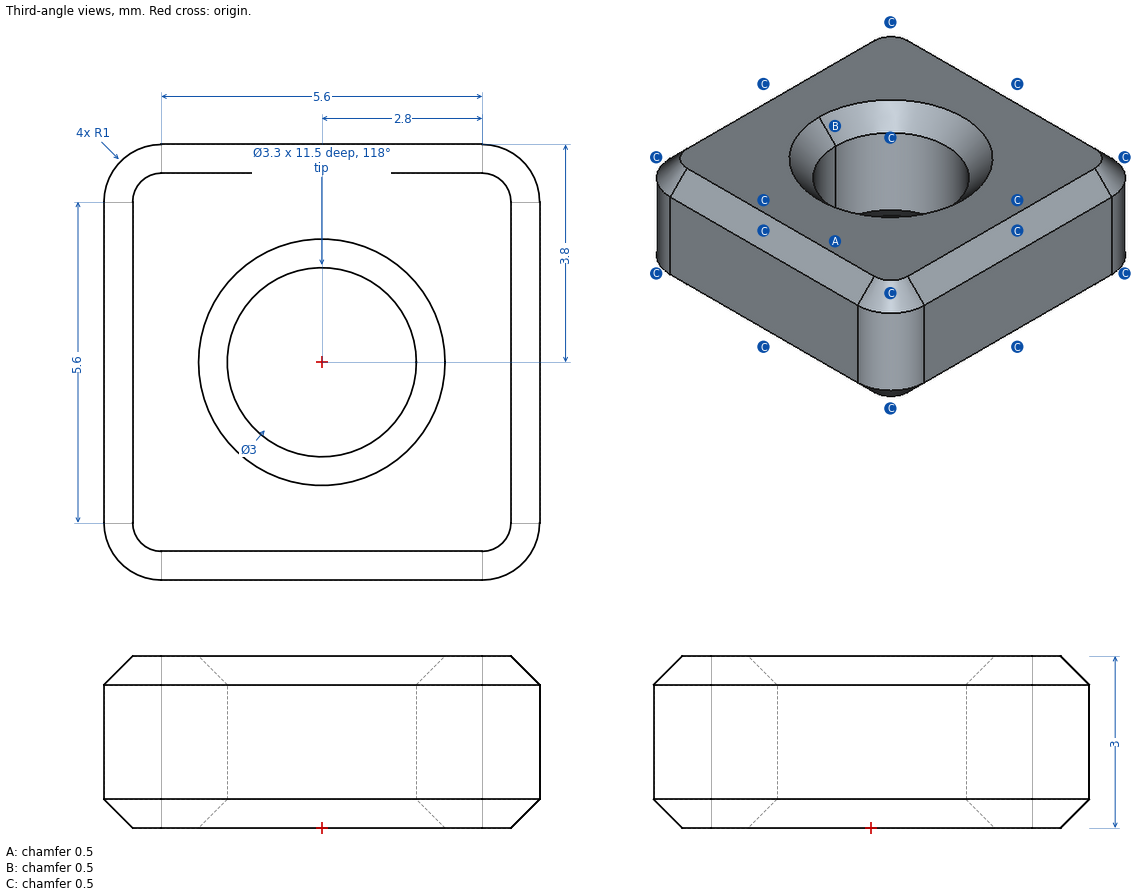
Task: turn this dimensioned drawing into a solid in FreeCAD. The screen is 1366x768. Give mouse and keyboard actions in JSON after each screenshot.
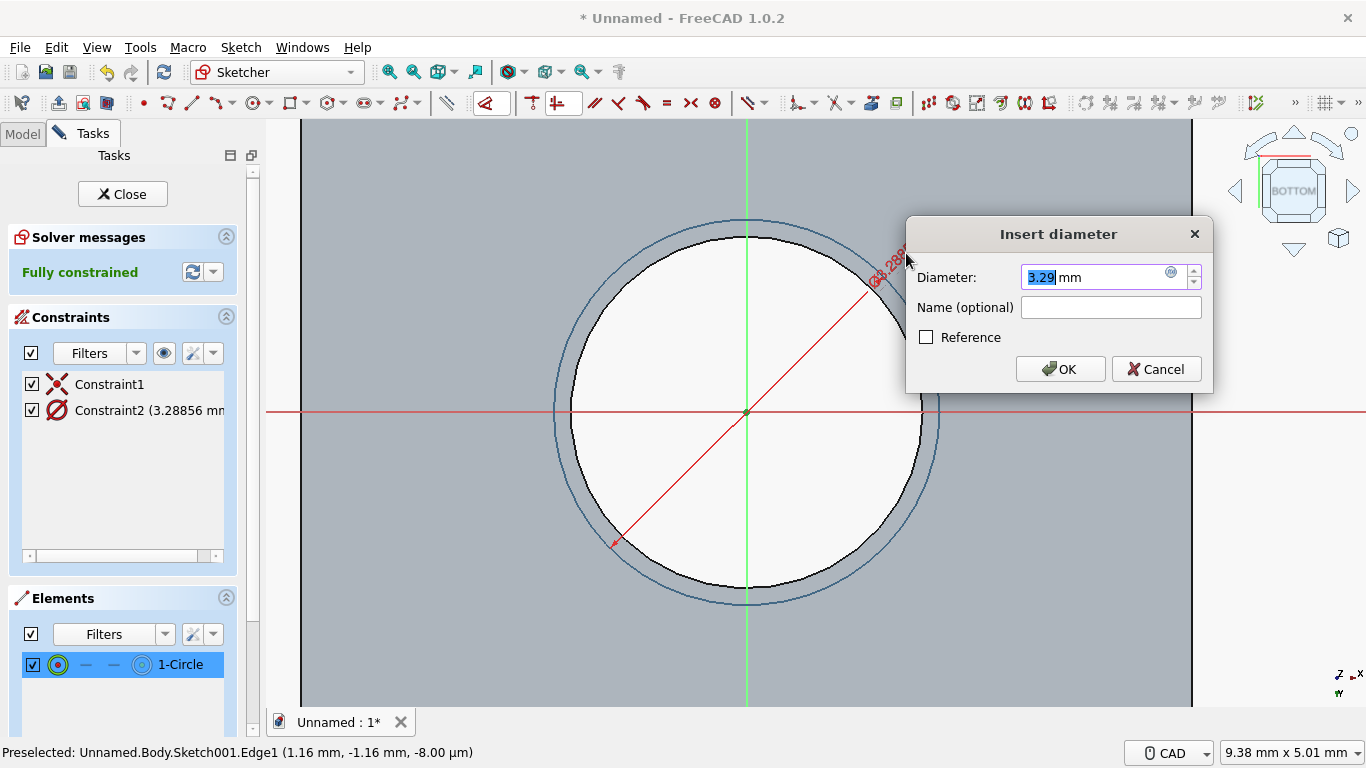
{"action": "type", "text": "3.3"}
{"action": "key", "text": "Return"}
{"action": "key", "text": "Escape"}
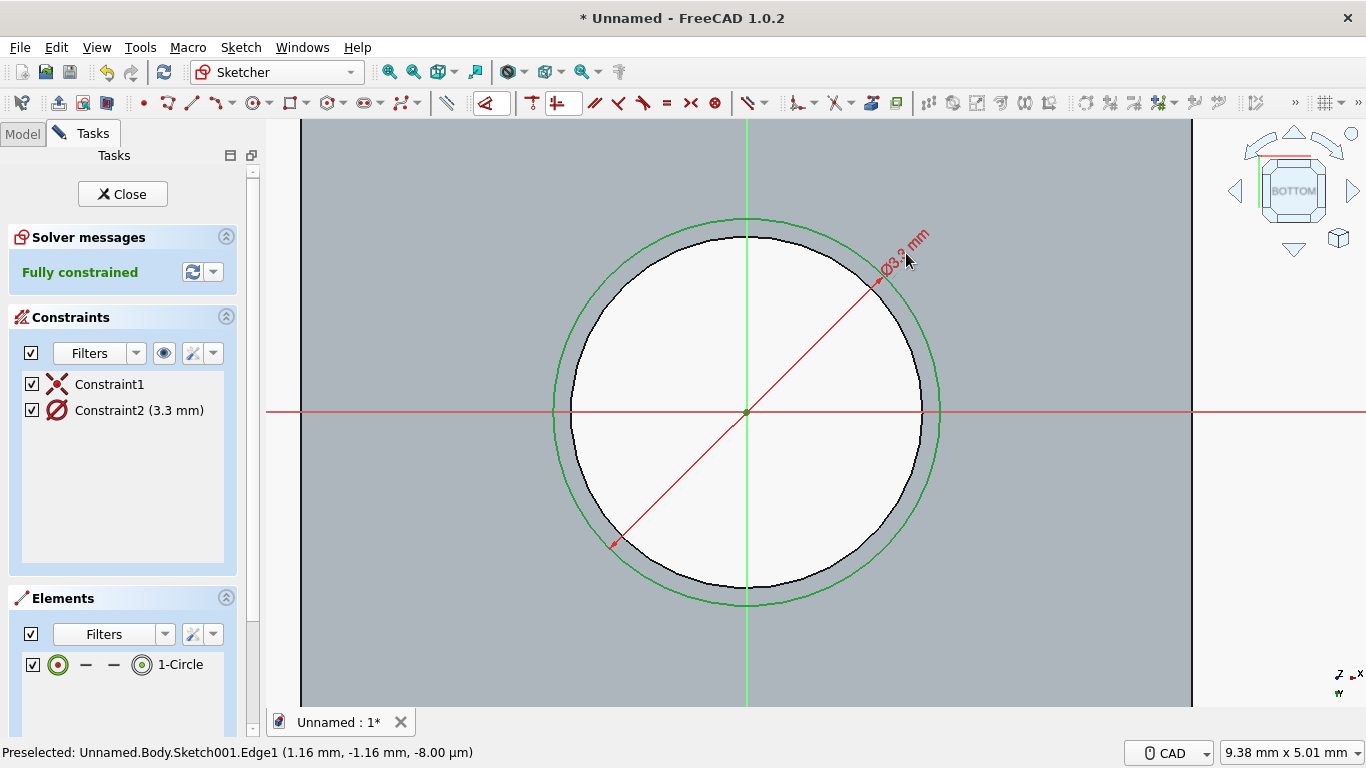
{"action": "left_click", "coordinate": [123, 194]}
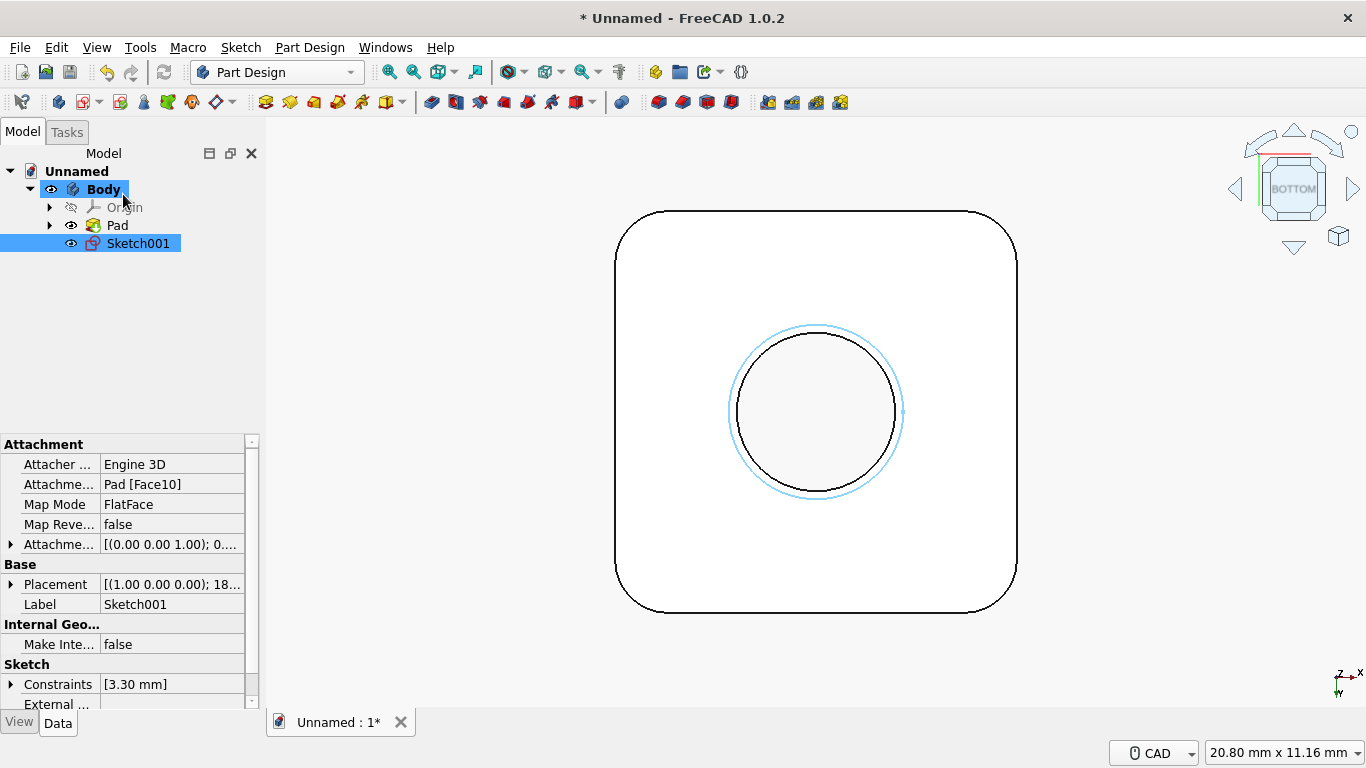
{"action": "left_click", "coordinate": [456, 102]}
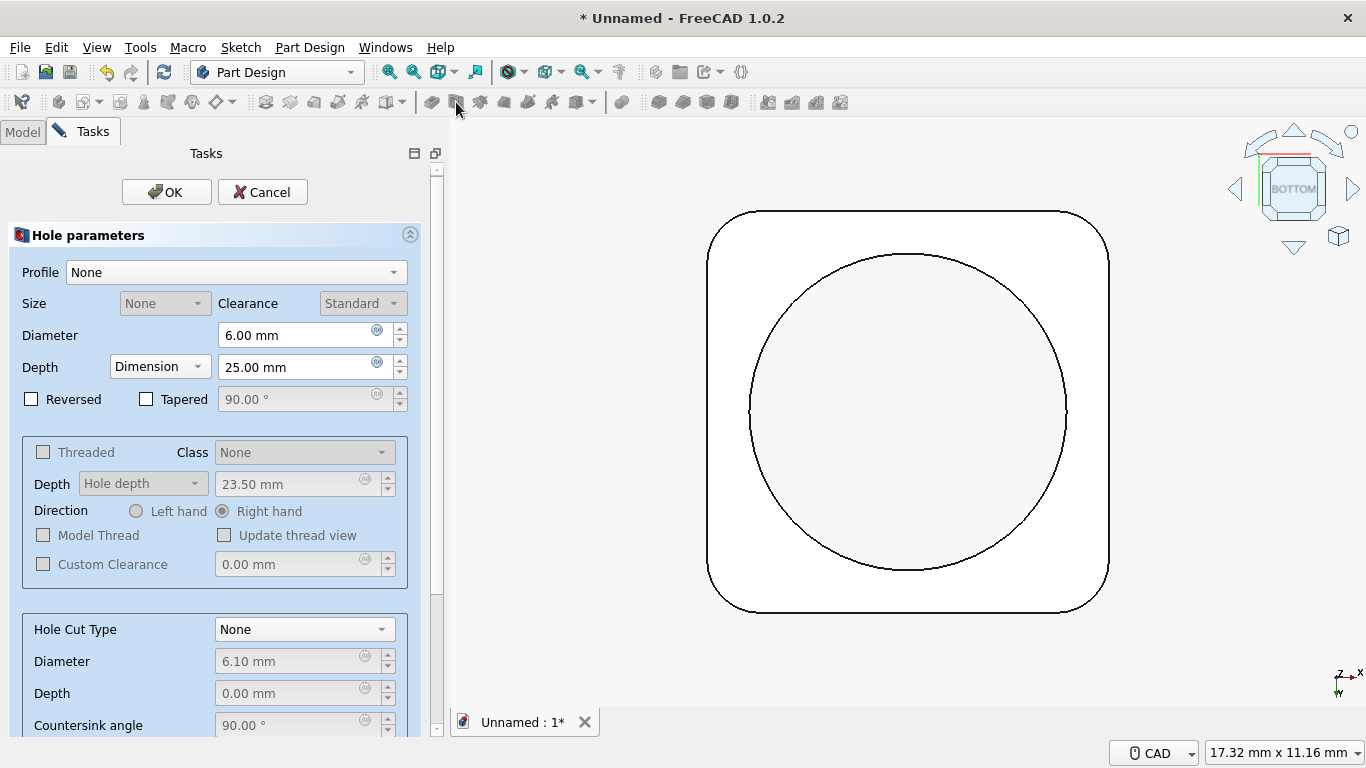
{"action": "triple_click", "coordinate": [305, 335]}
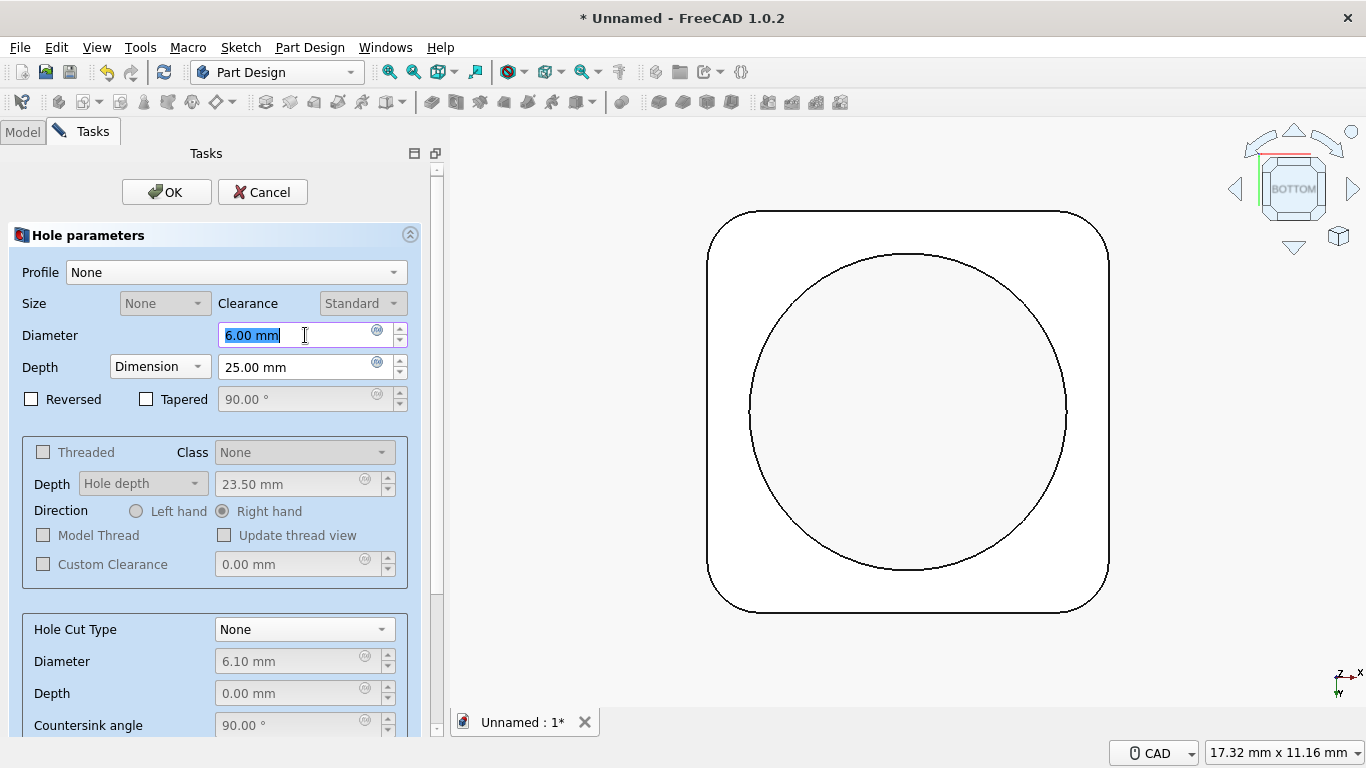
{"action": "type", "text": "3.3"}
{"action": "key", "text": "Tab"}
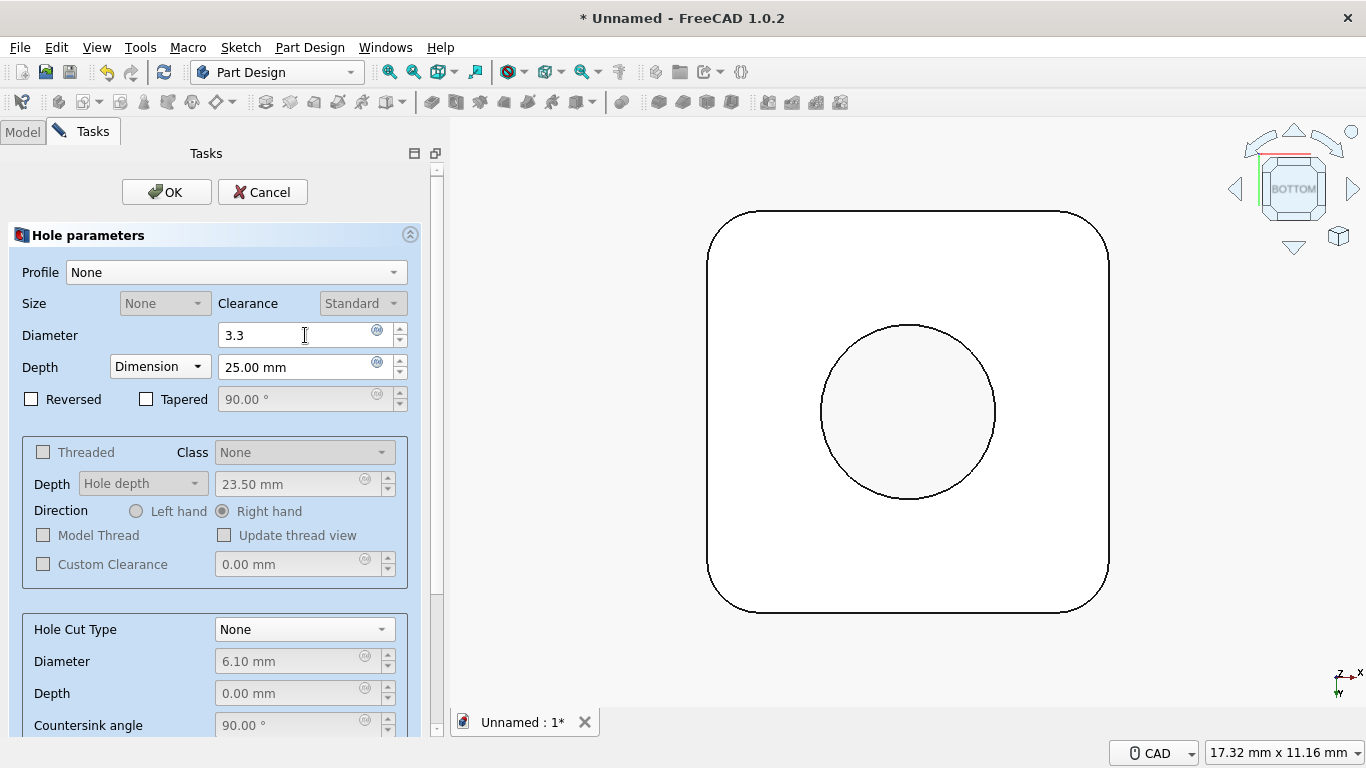
{"action": "triple_click", "coordinate": [305, 367]}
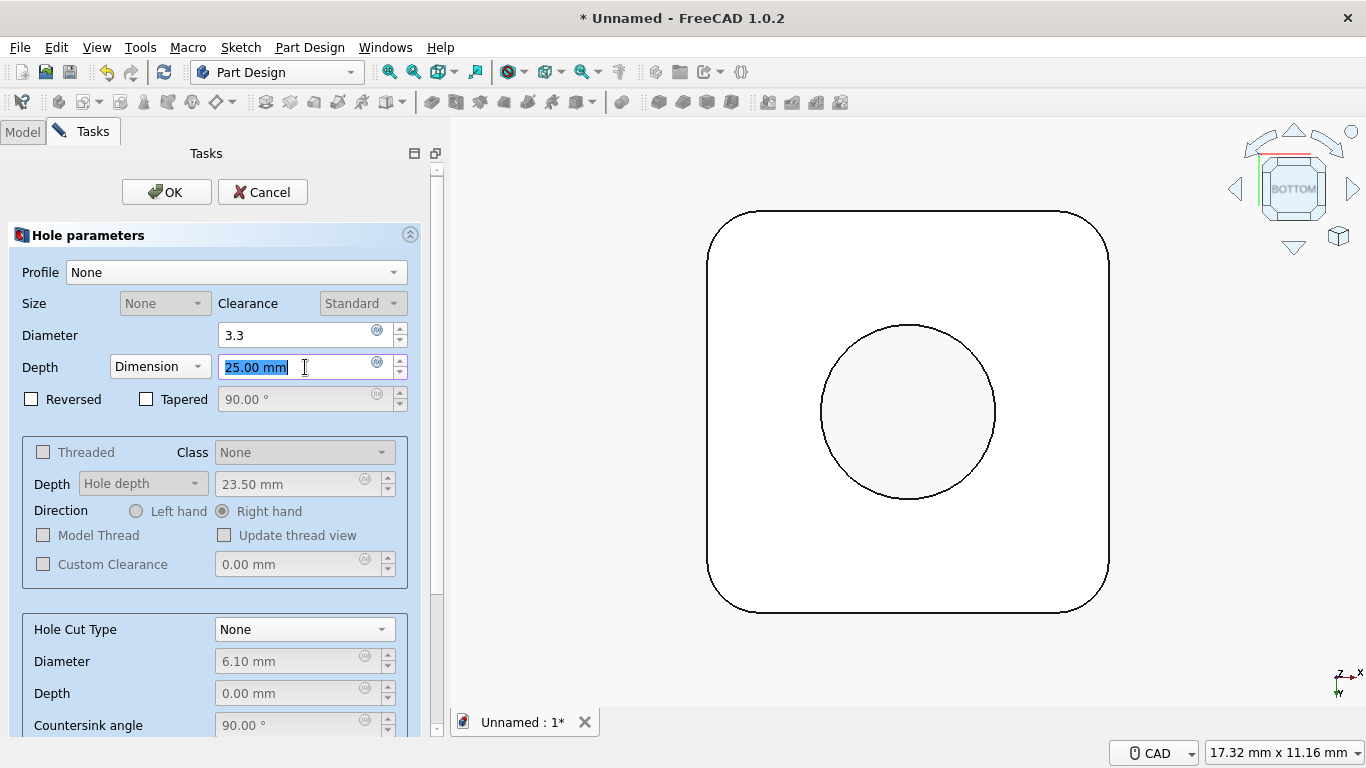
{"action": "type", "text": "11.5"}
{"action": "key", "text": "Tab"}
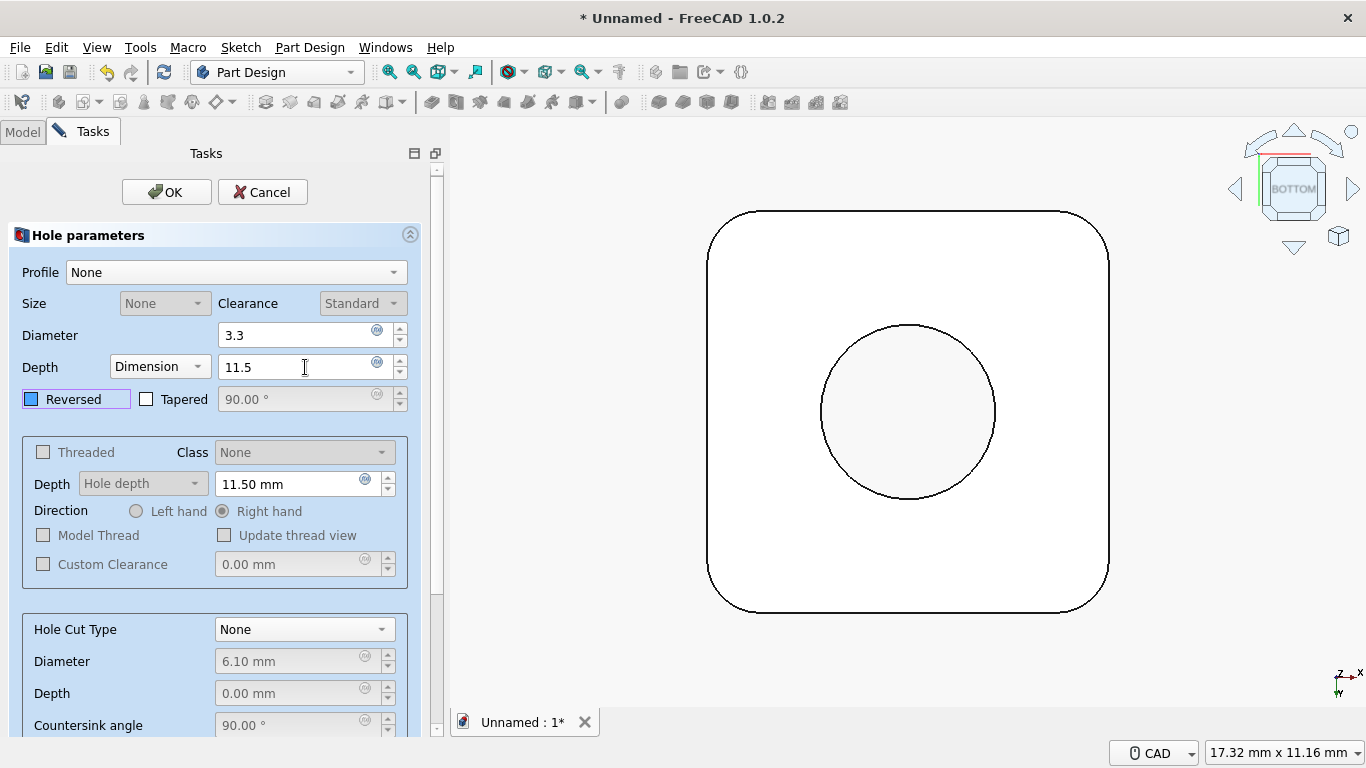
{"action": "left_click", "coordinate": [167, 192]}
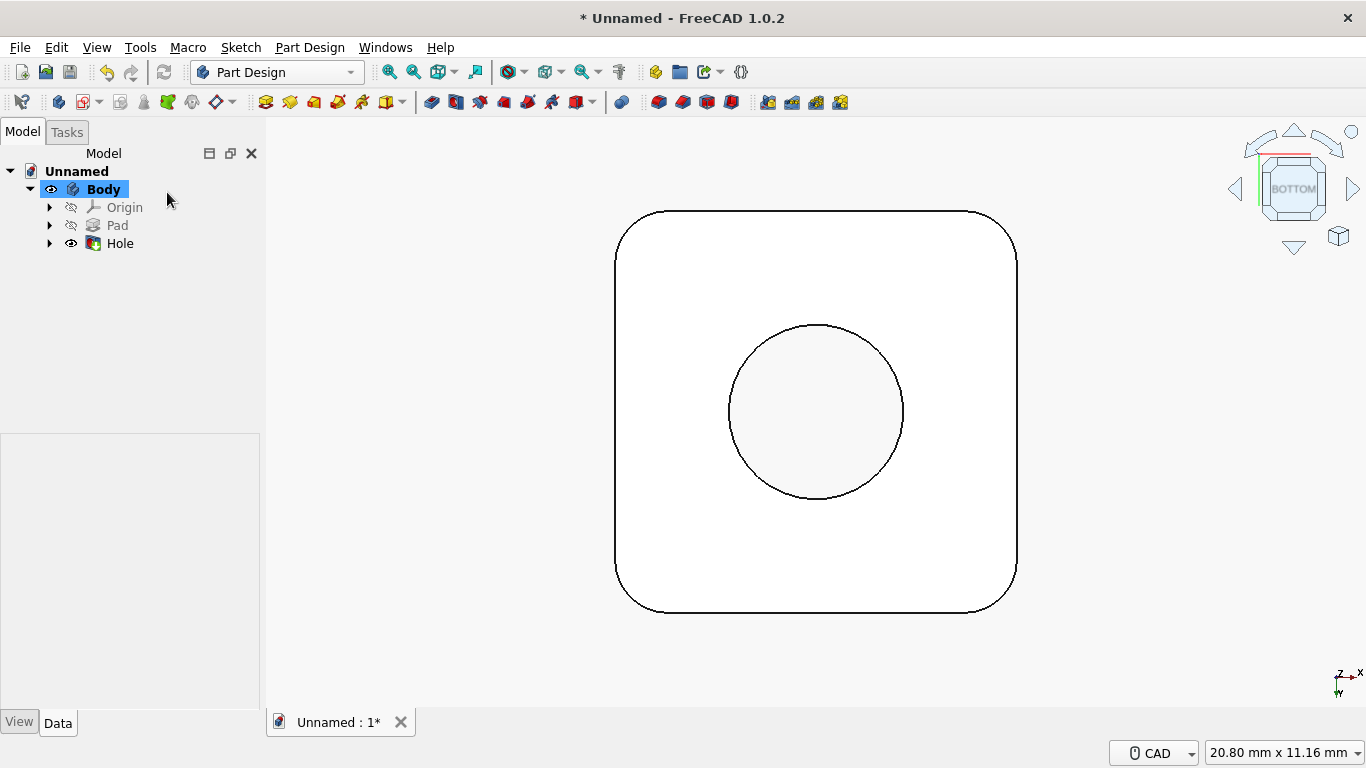
{"action": "left_click", "coordinate": [903, 411]}